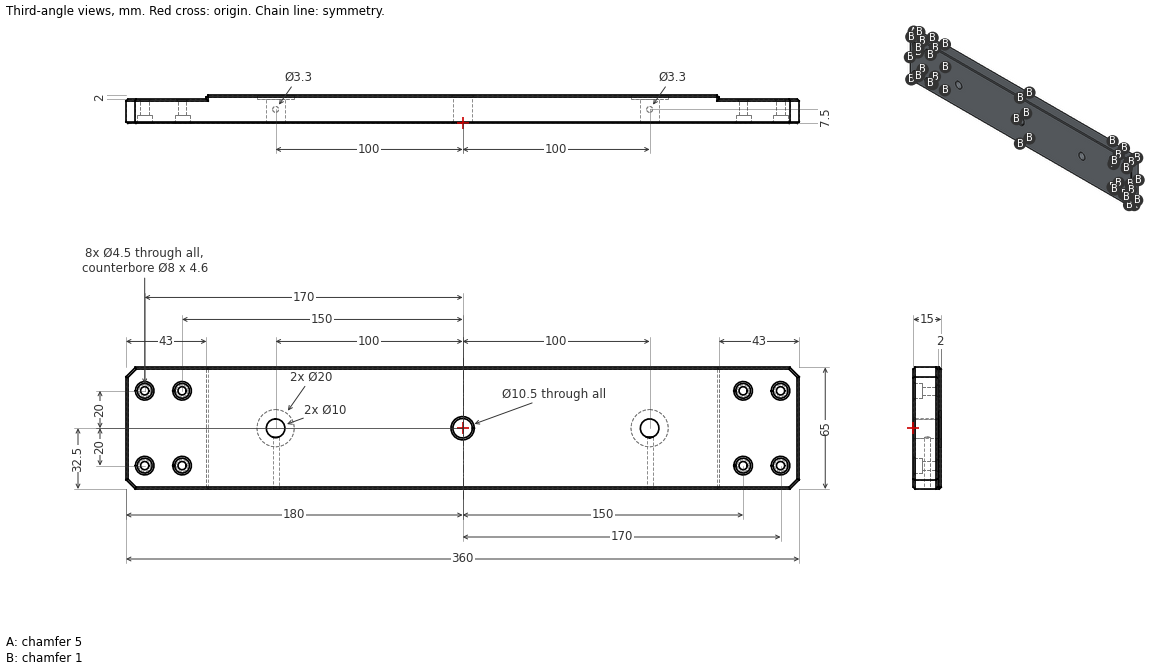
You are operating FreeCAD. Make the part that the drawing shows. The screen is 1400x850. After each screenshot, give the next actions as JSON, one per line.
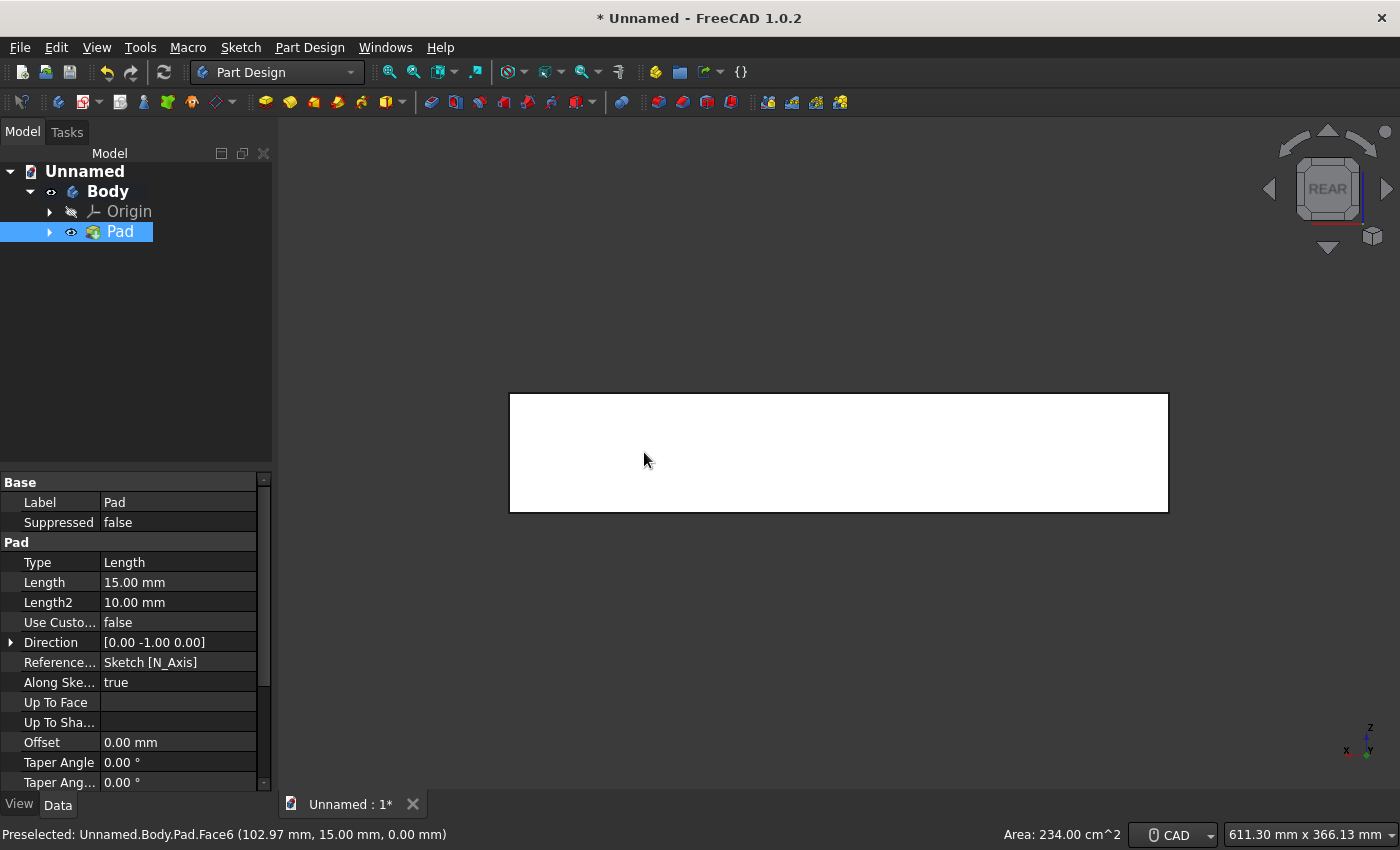
{"action": "left_click", "coordinate": [84, 102]}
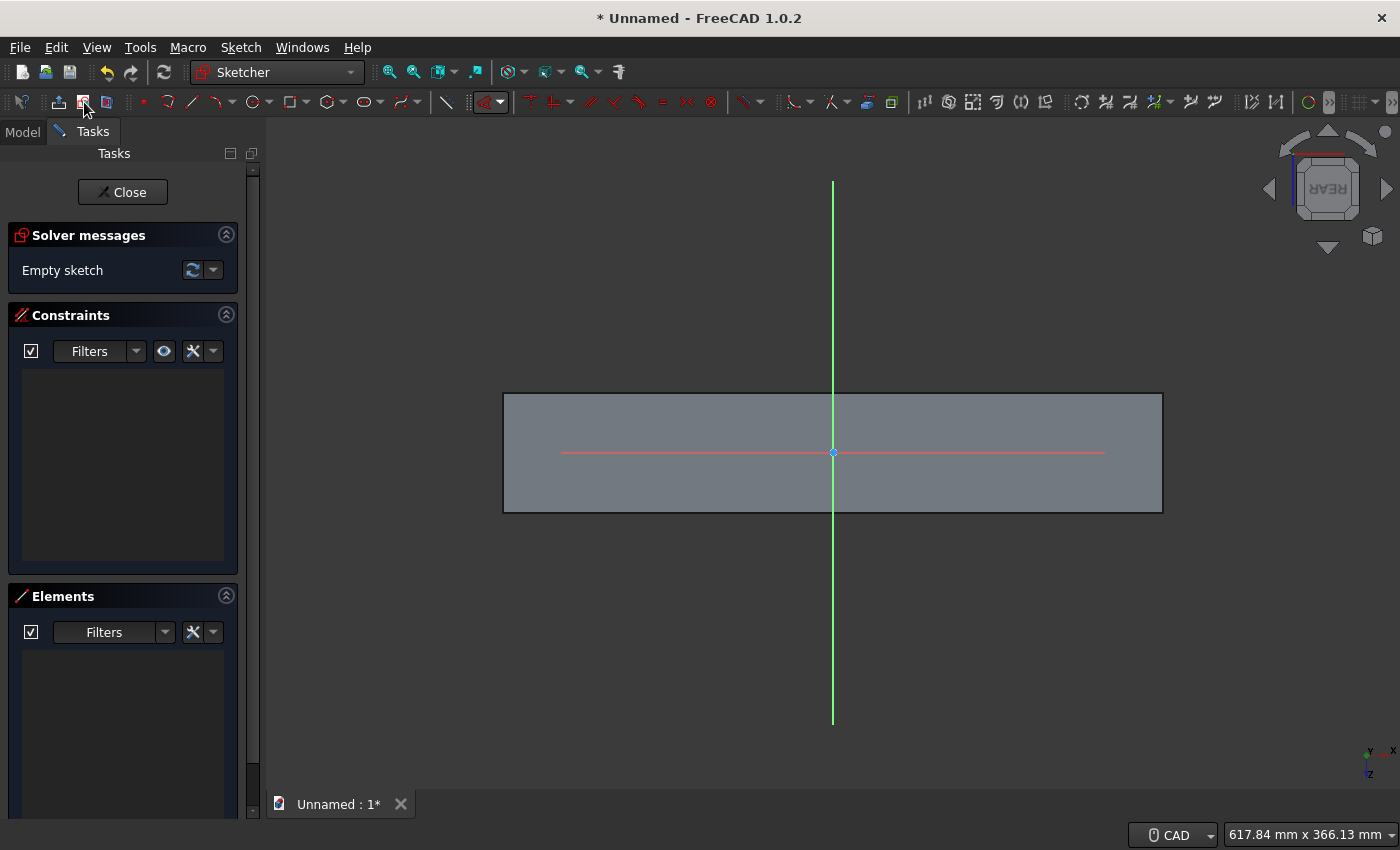
{"action": "key", "text": "g r"}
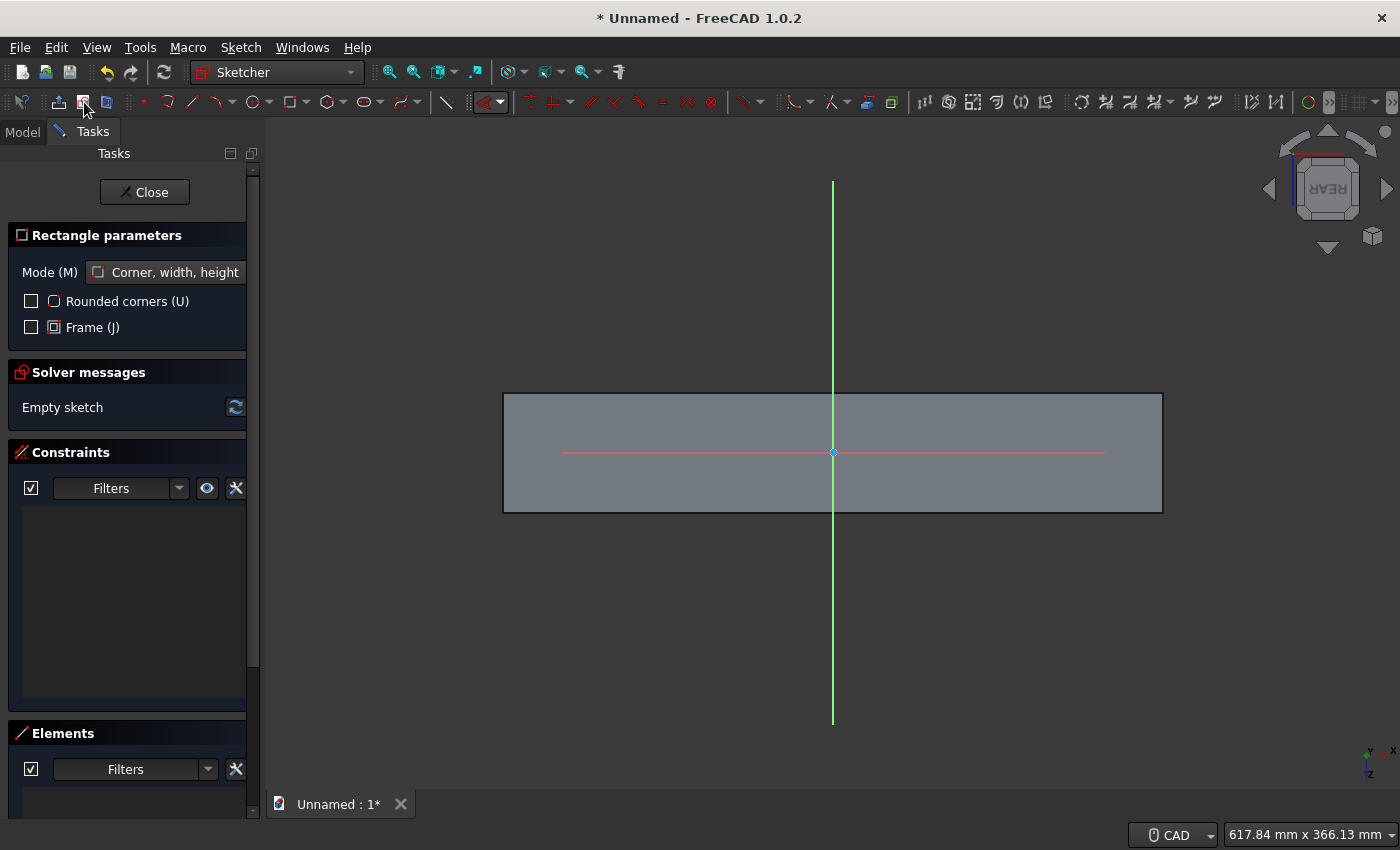
{"action": "left_click", "coordinate": [503, 393]}
{"action": "mouse_move", "coordinate": [582, 513]}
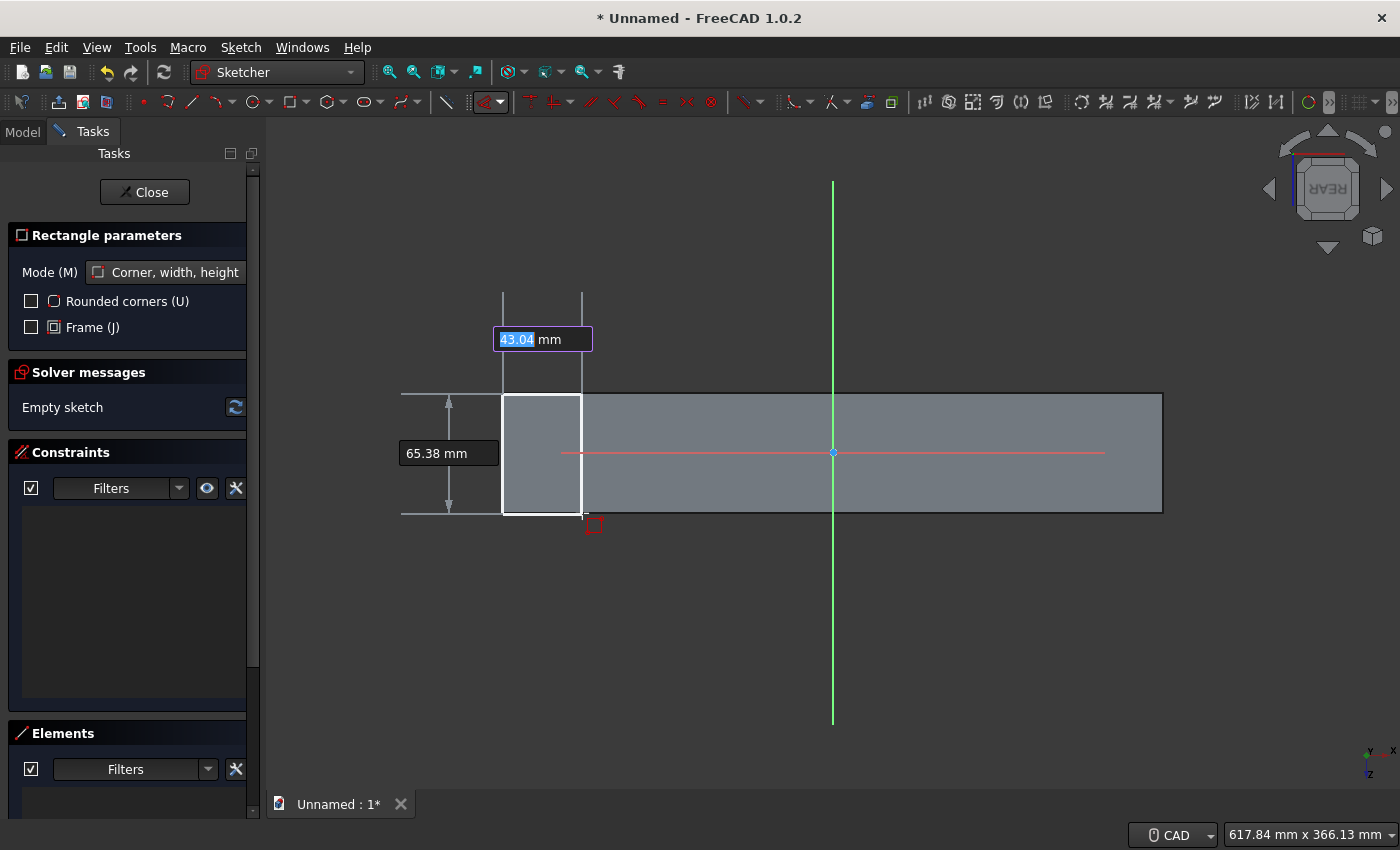
{"action": "type", "text": "43"}
{"action": "key", "text": "Tab"}
{"action": "type", "text": "65"}
{"action": "key", "text": "Return"}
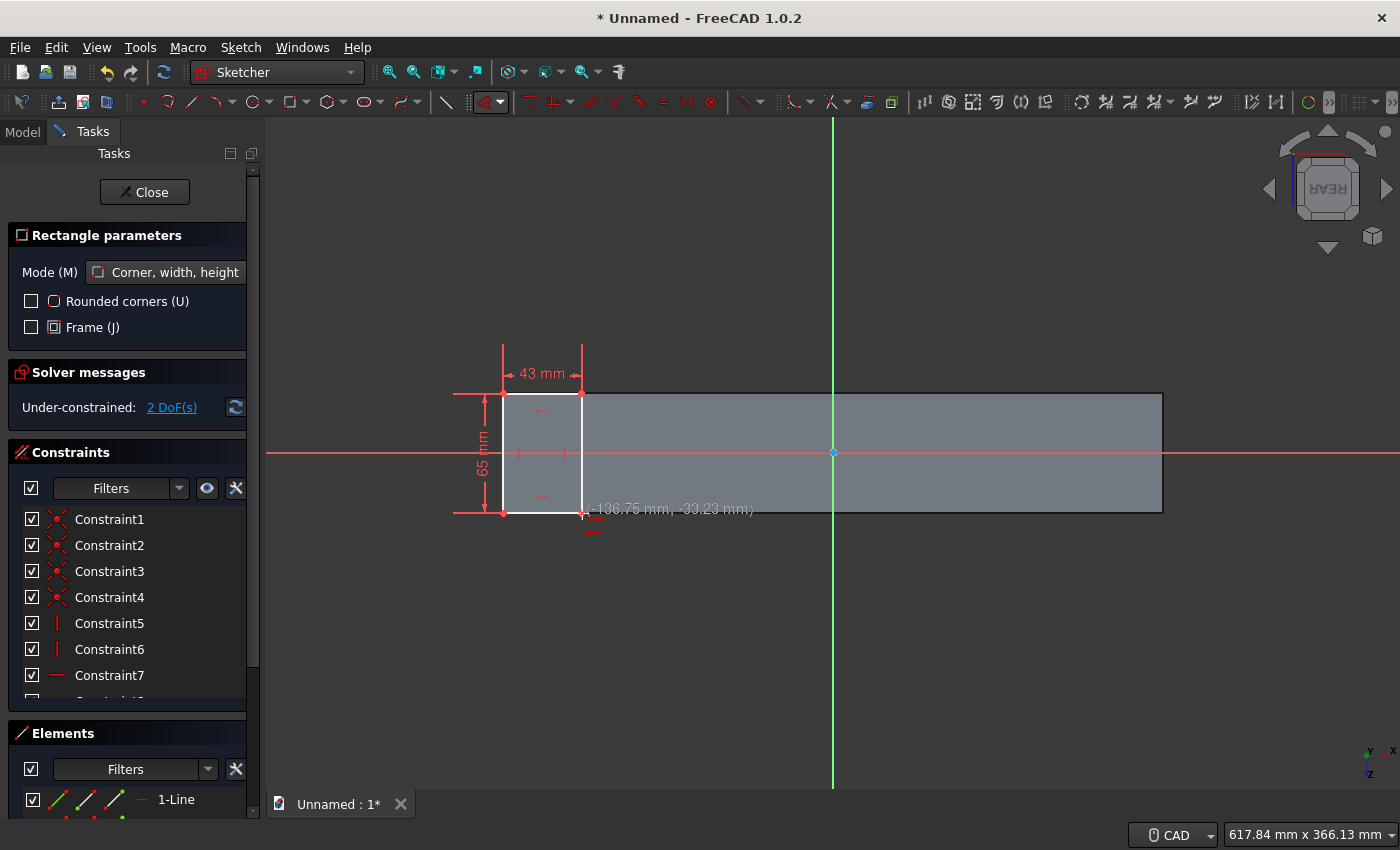
{"action": "left_click", "coordinate": [1084, 393]}
{"action": "mouse_move", "coordinate": [1163, 513]}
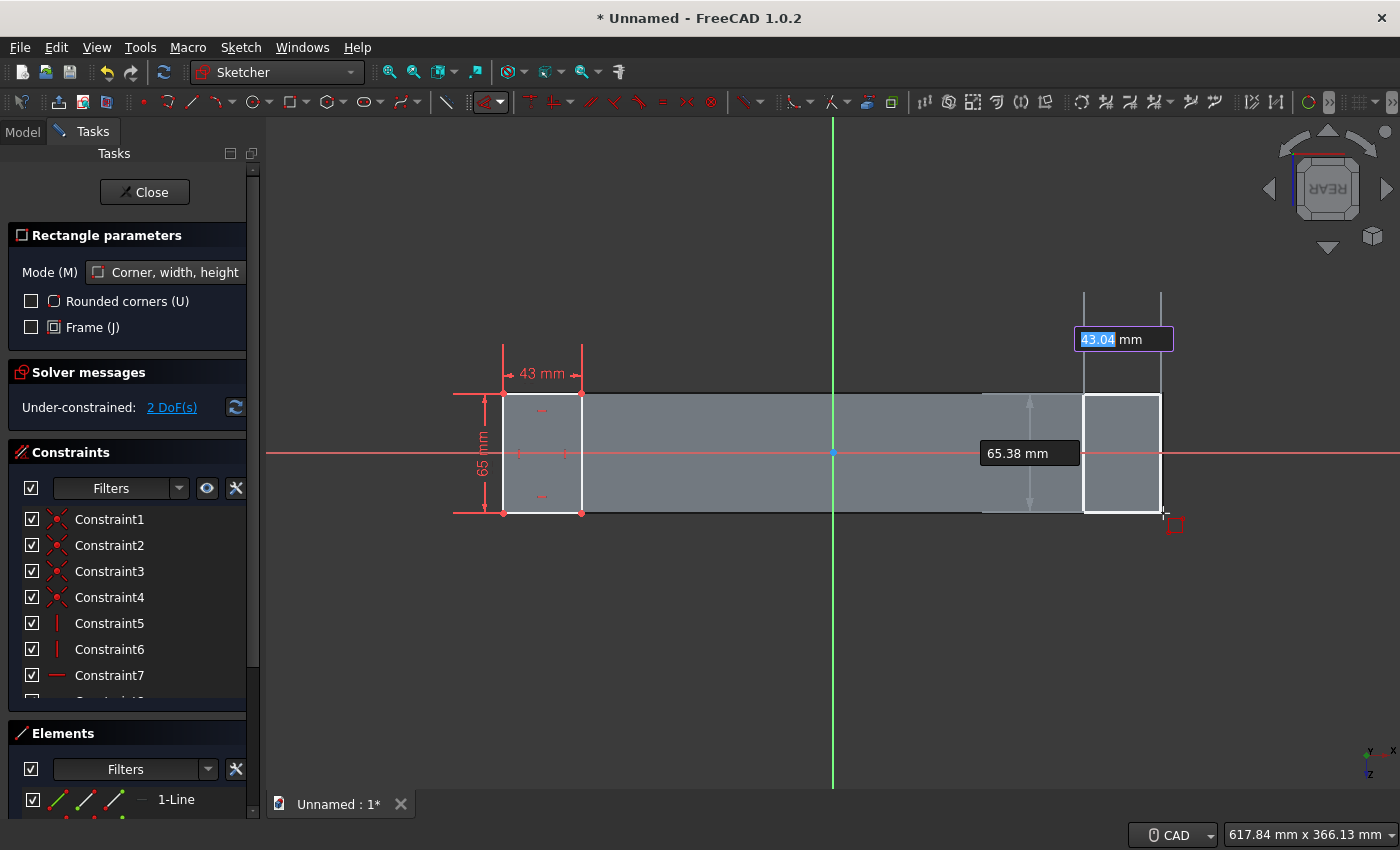
{"action": "type", "text": "43"}
{"action": "key", "text": "Tab"}
{"action": "type", "text": "65"}
{"action": "key", "text": "Return"}
{"action": "key", "text": "Escape"}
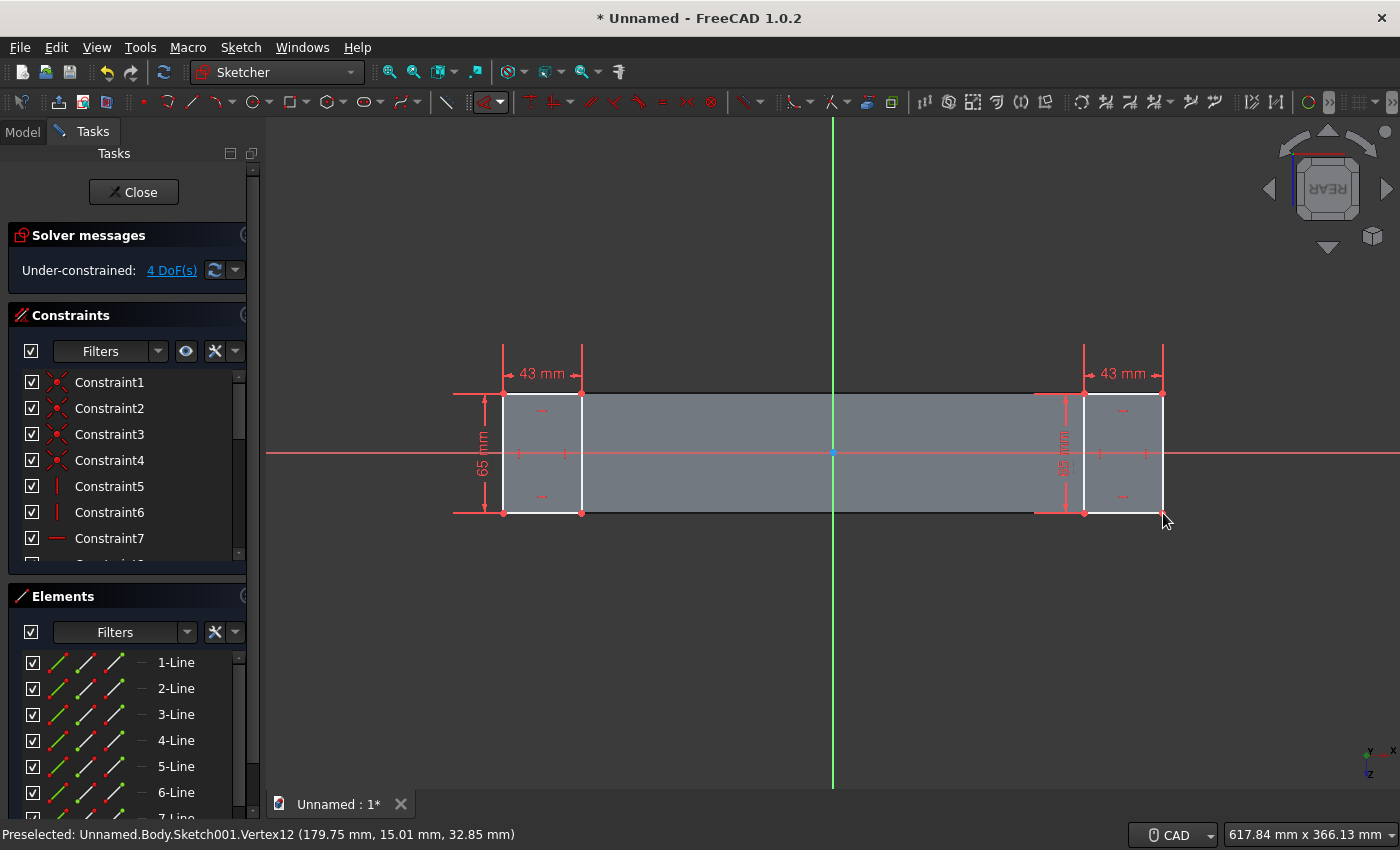
{"action": "left_click", "coordinate": [582, 394]}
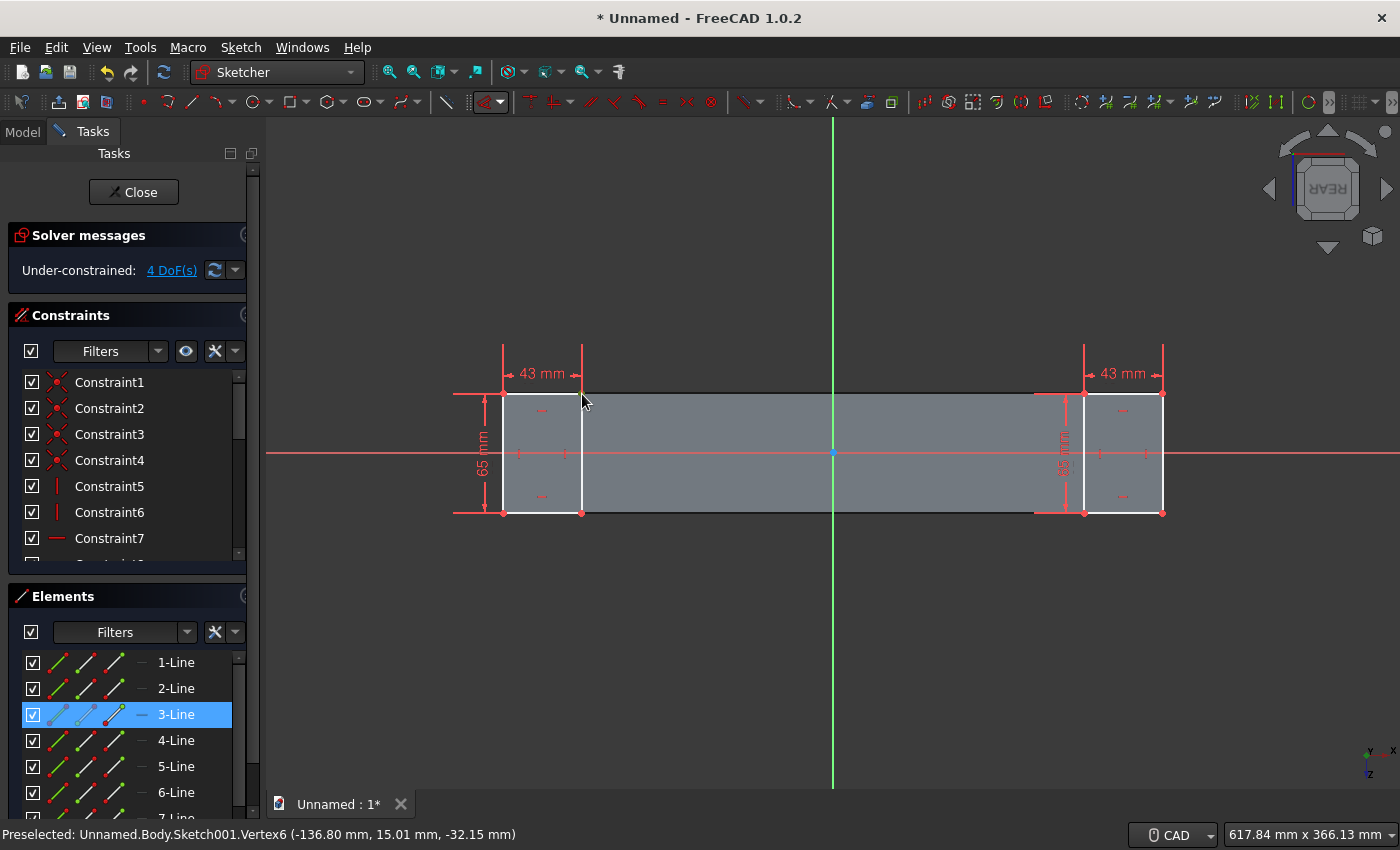
{"action": "left_click", "coordinate": [1084, 394]}